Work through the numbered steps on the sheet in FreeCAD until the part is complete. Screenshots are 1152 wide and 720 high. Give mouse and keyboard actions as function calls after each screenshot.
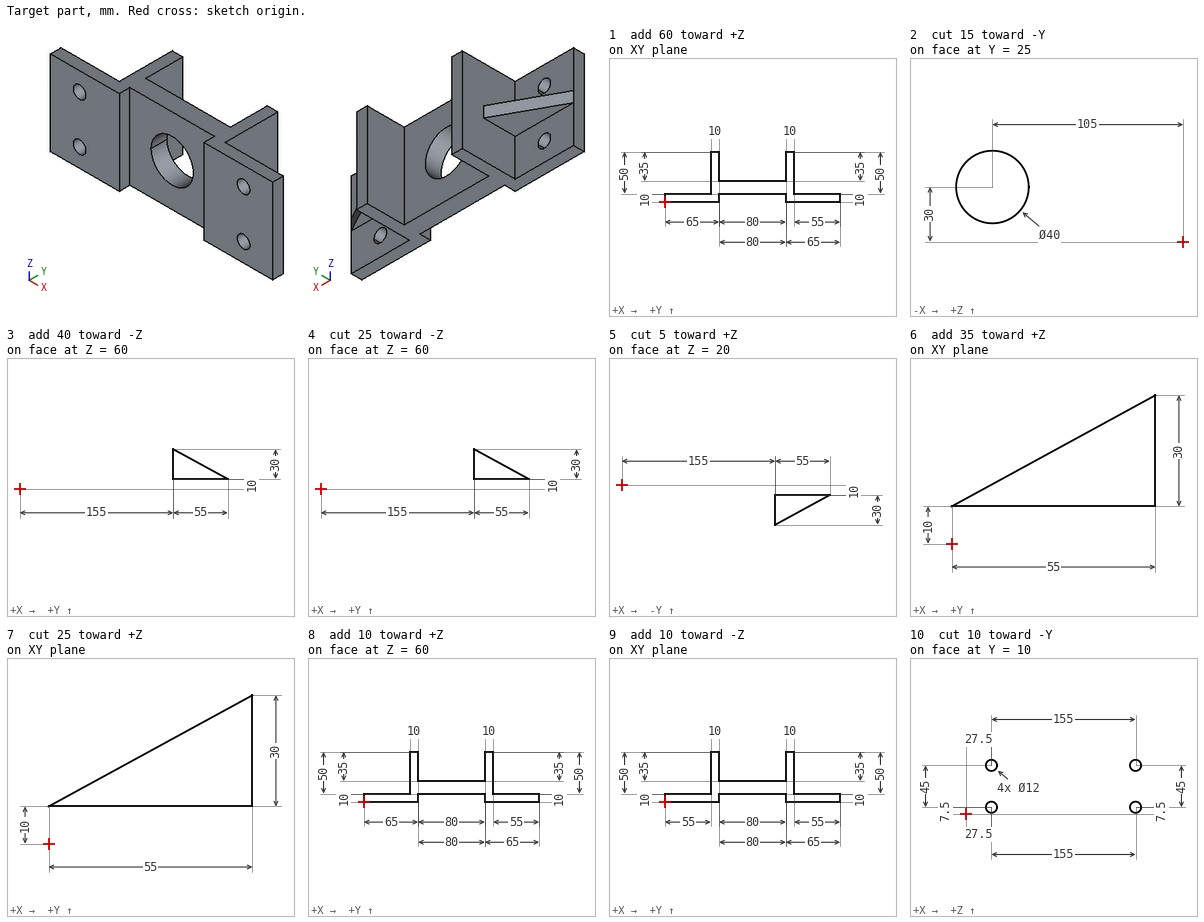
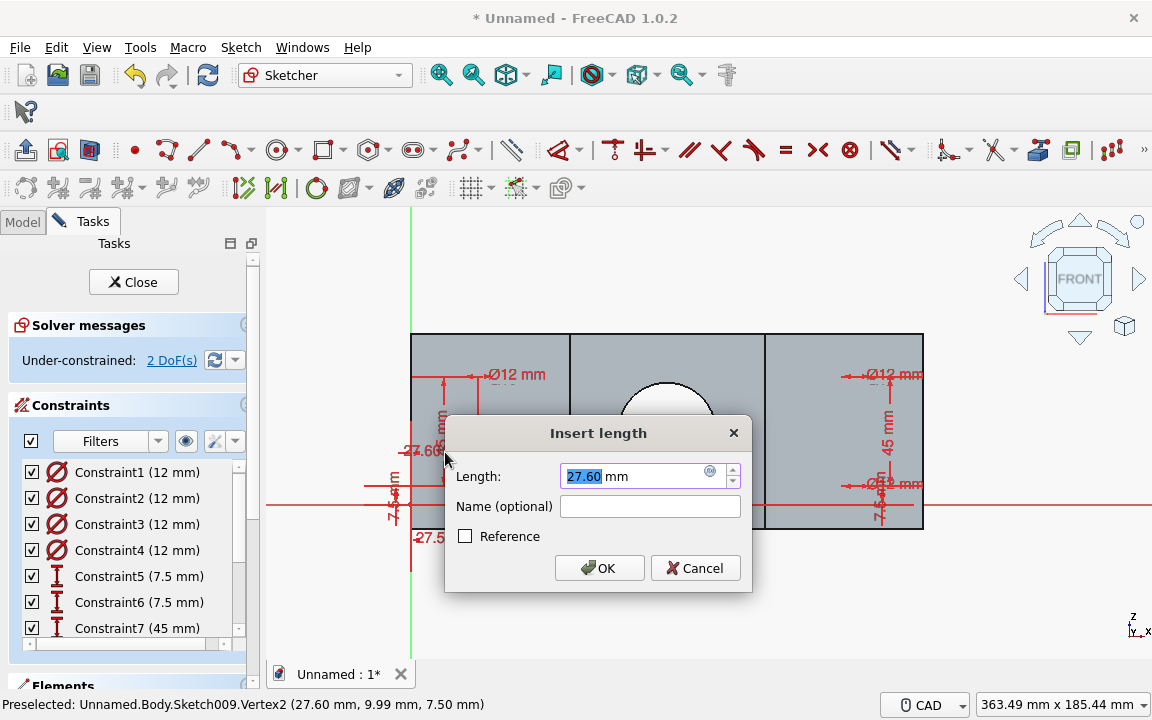
text(27.5)
key(Return)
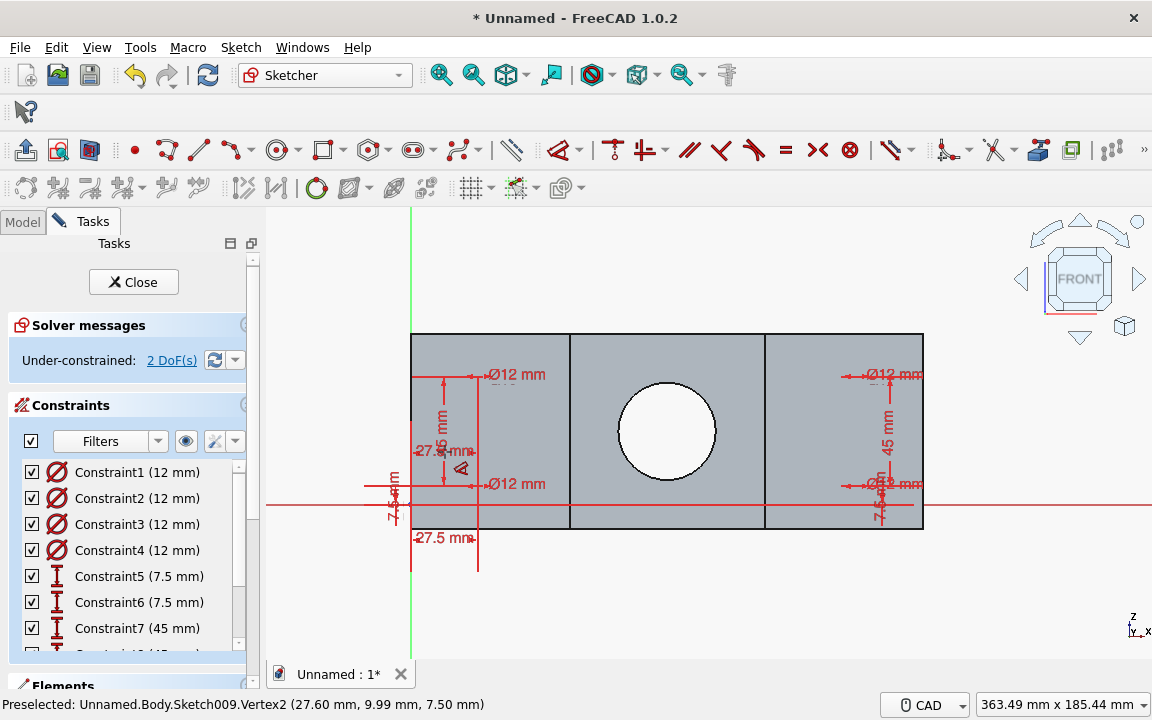
click(478, 486)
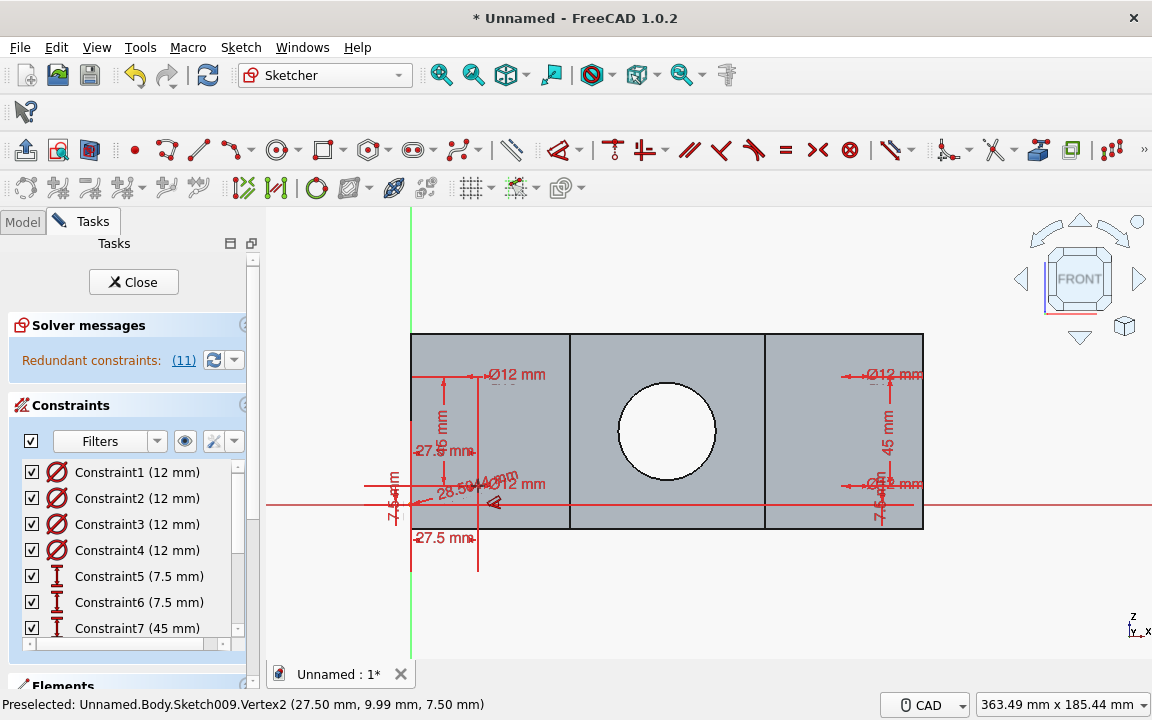
click(856, 486)
click(667, 520)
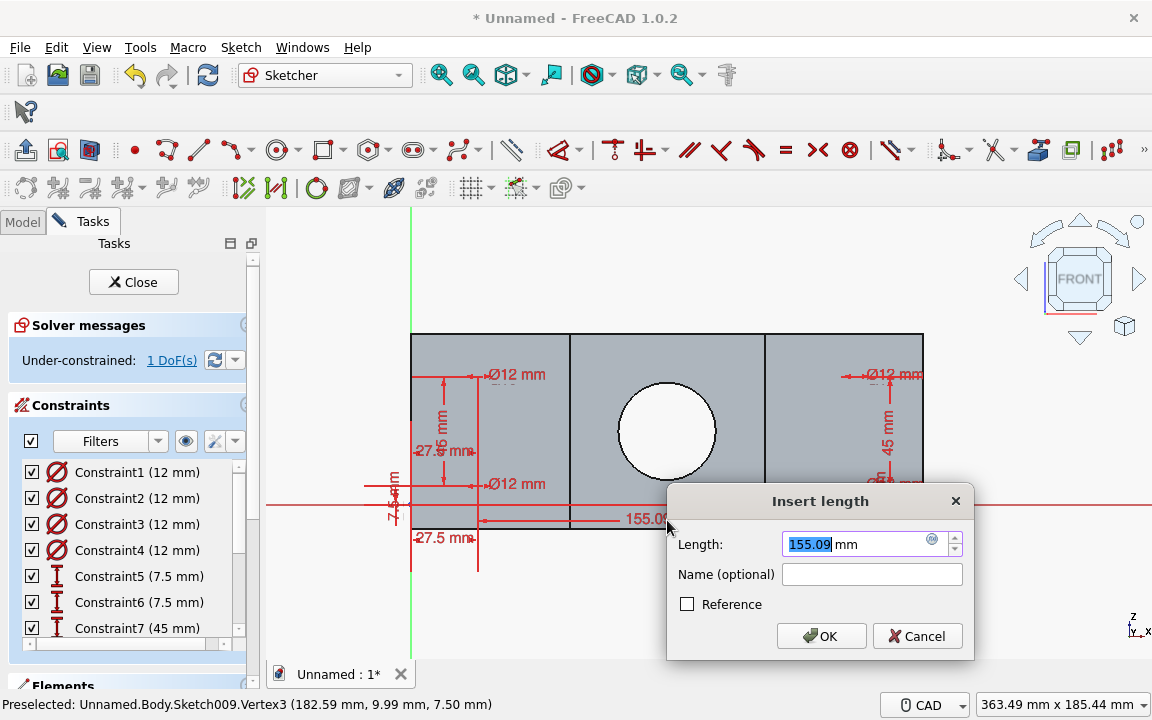
text(155)
key(Return)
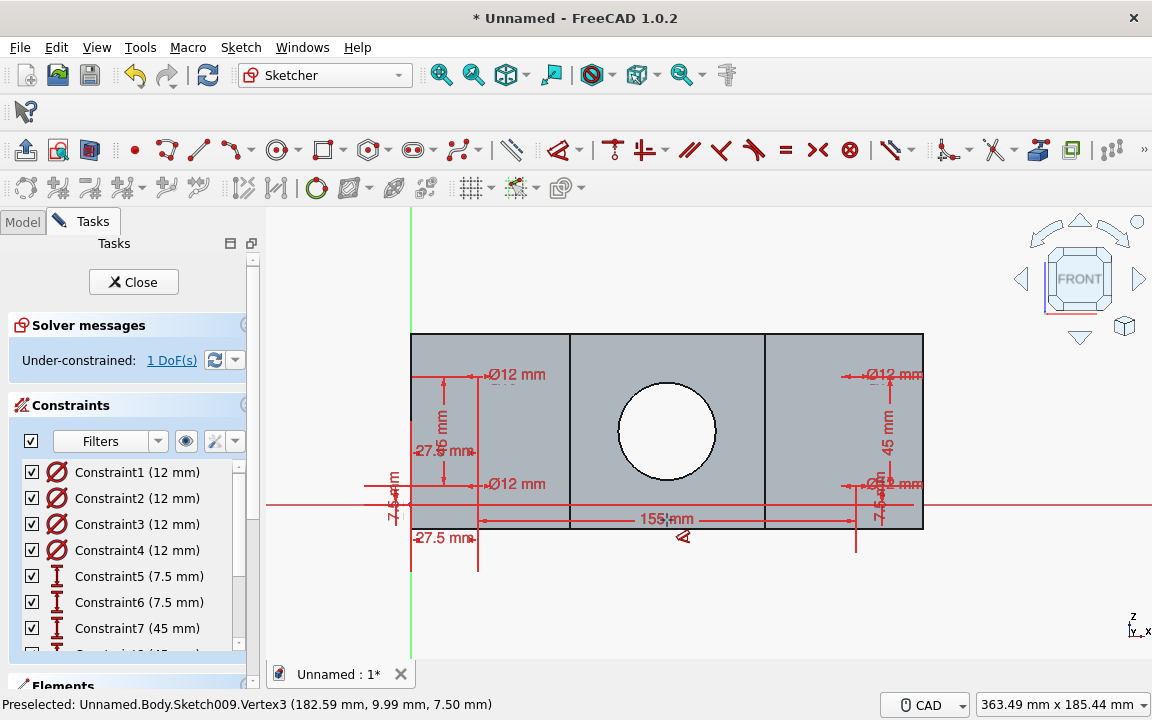
click(478, 377)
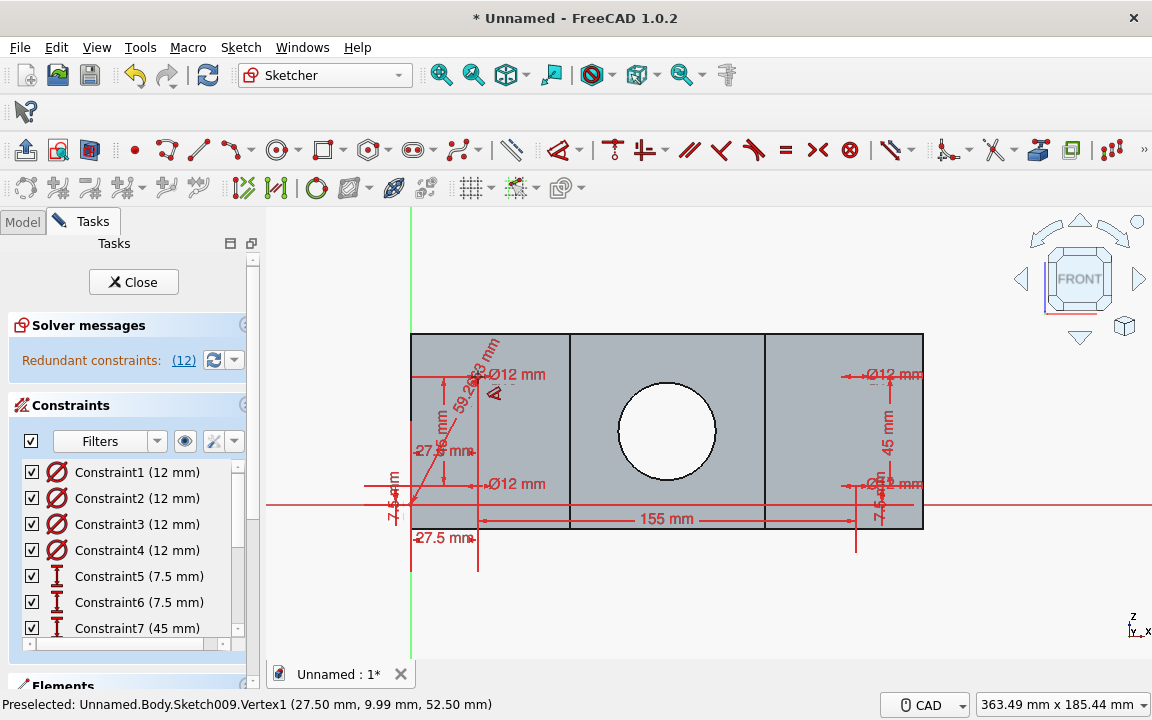
click(856, 377)
click(667, 343)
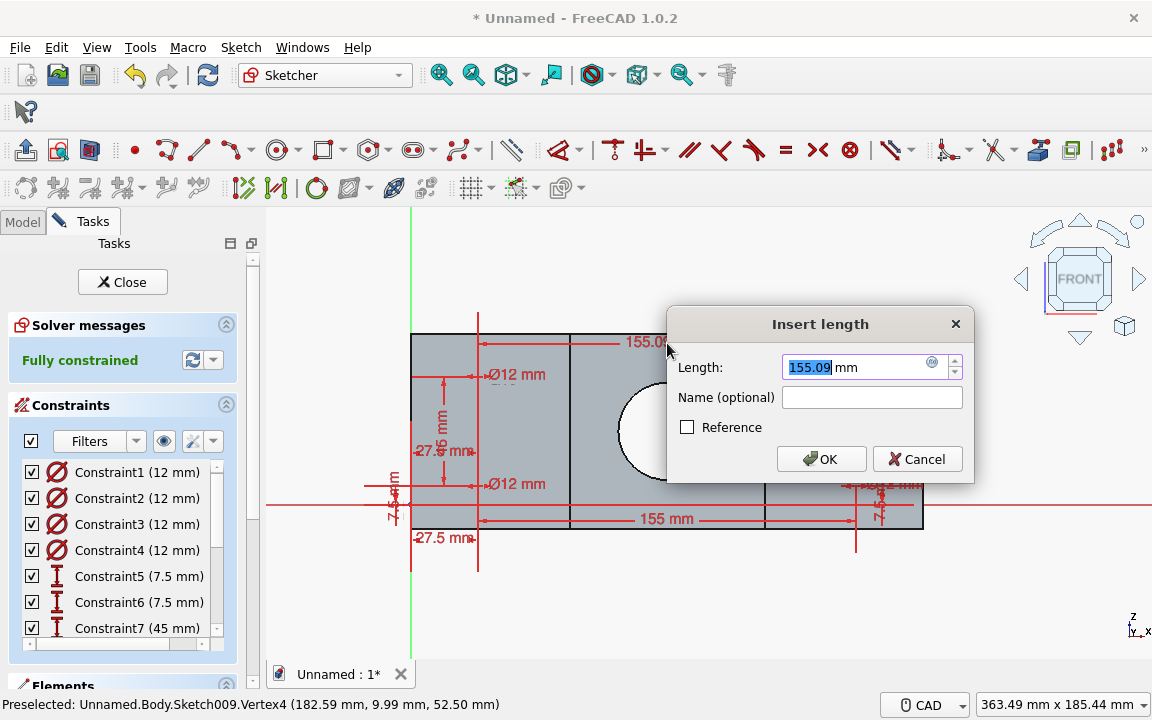
text(155)
key(Return)
key(Escape)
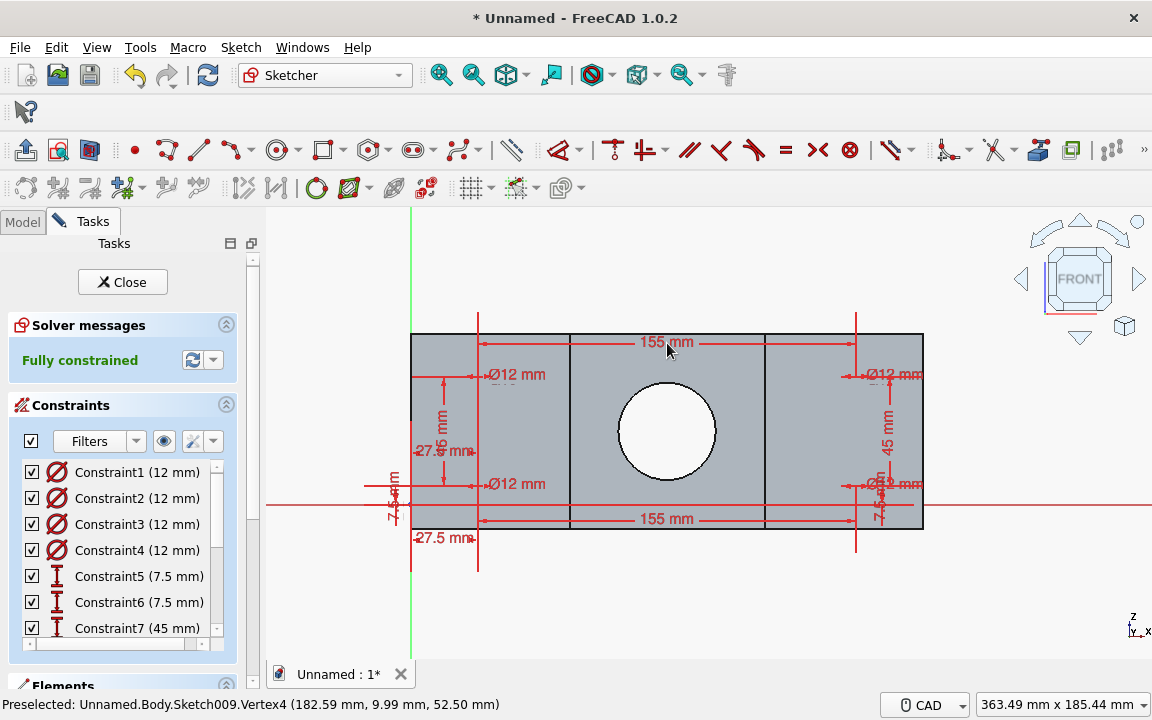
click(123, 282)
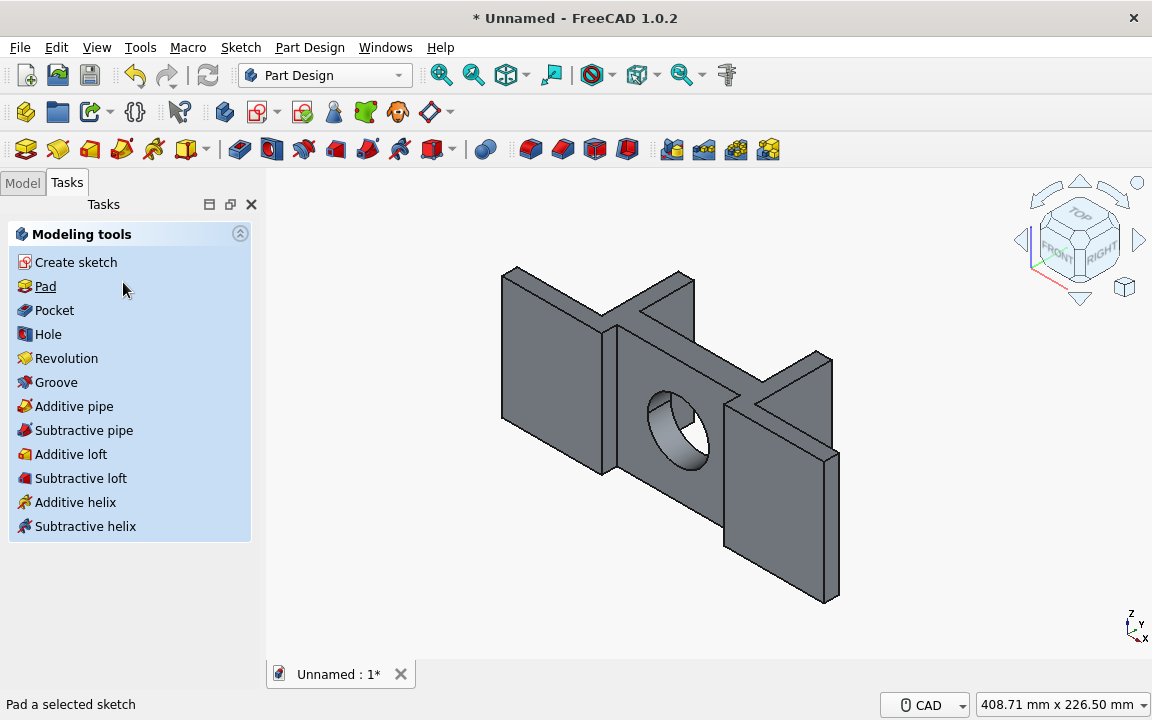
click(240, 150)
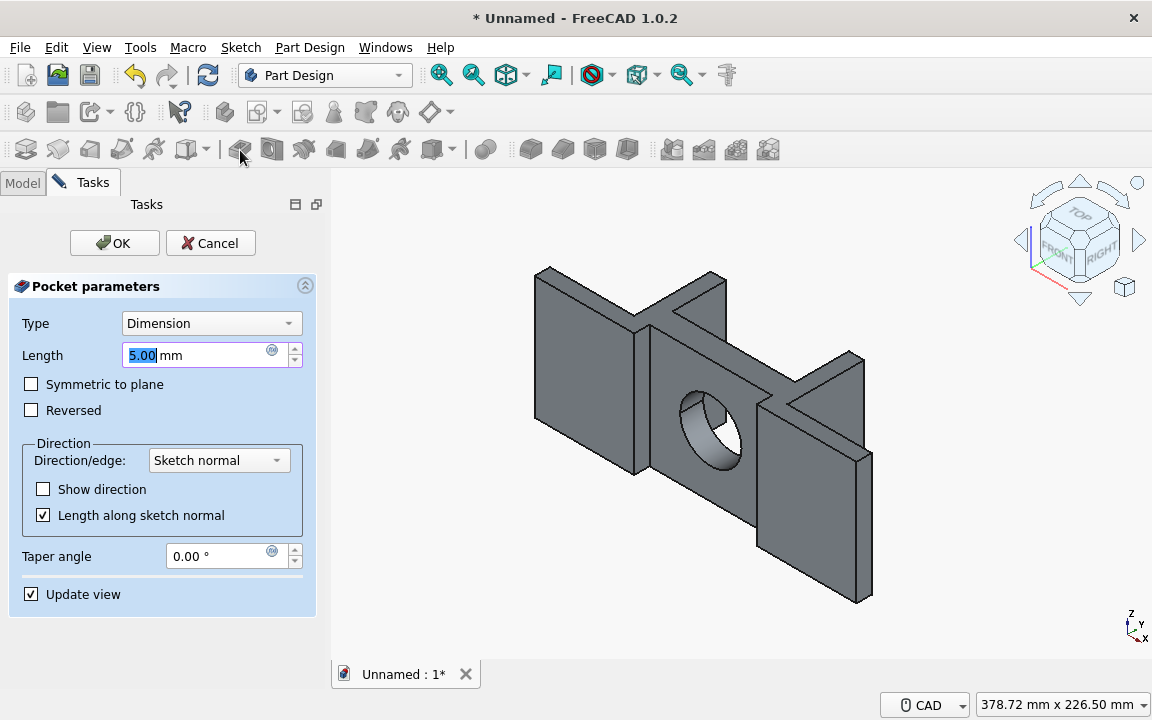
text(10)
key(Tab)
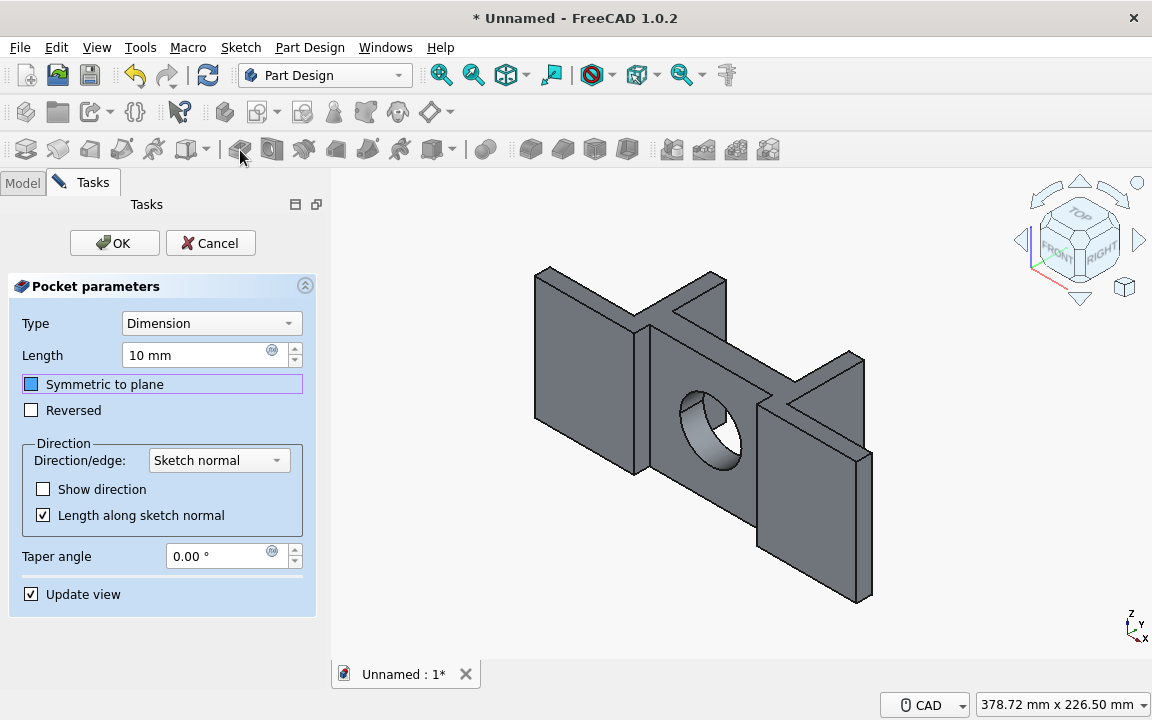
click(30, 410)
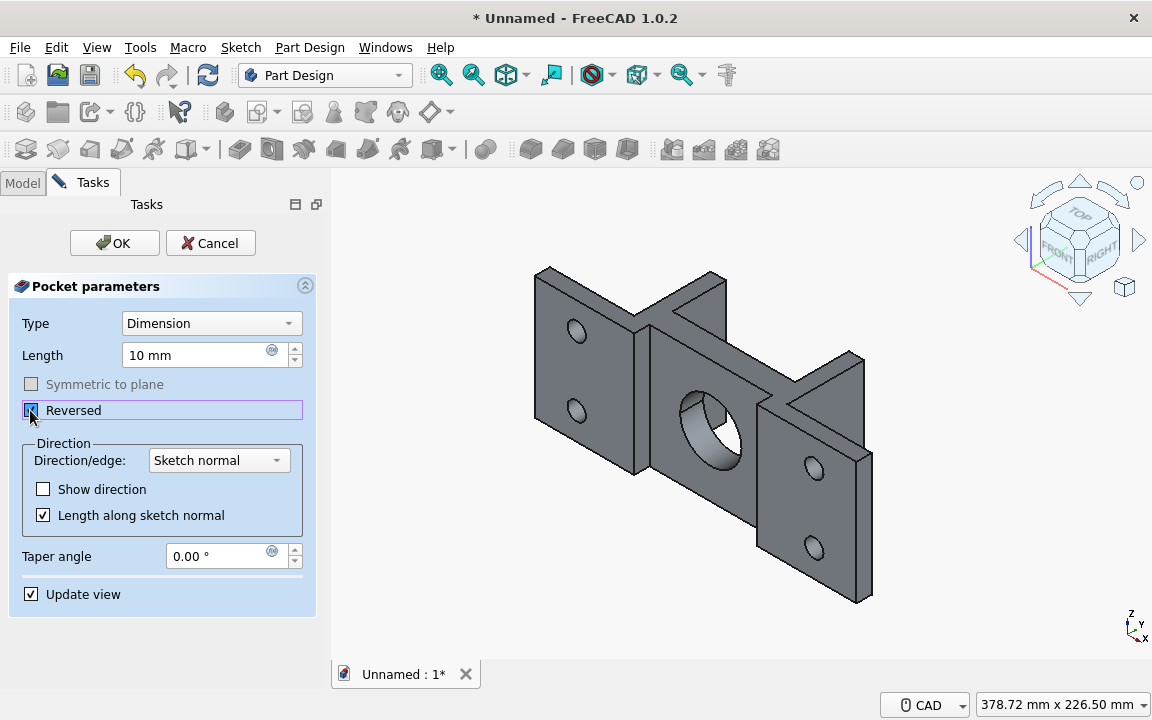
click(115, 243)